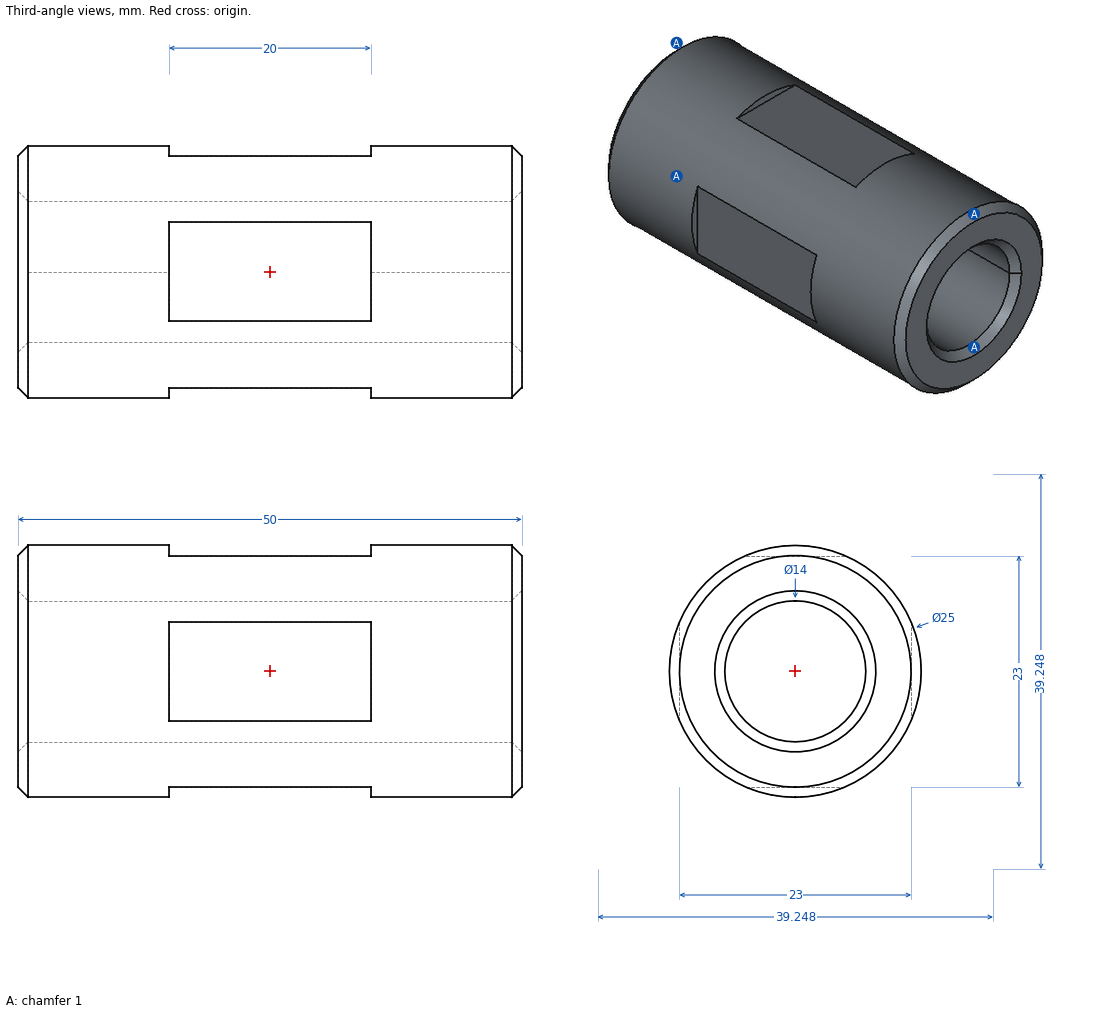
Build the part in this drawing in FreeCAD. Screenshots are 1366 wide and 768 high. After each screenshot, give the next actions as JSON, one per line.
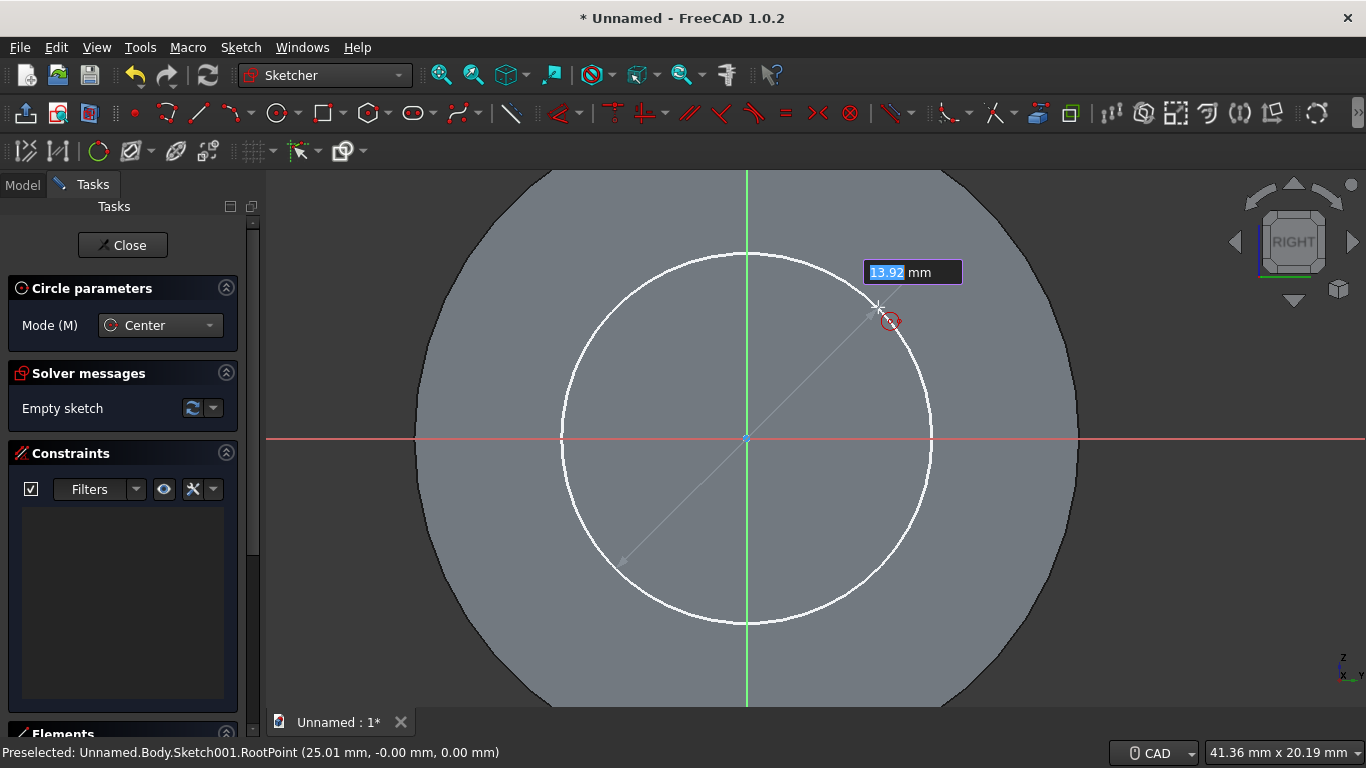
{"action": "type", "text": "14"}
{"action": "key", "text": "Return"}
{"action": "key", "text": "Escape"}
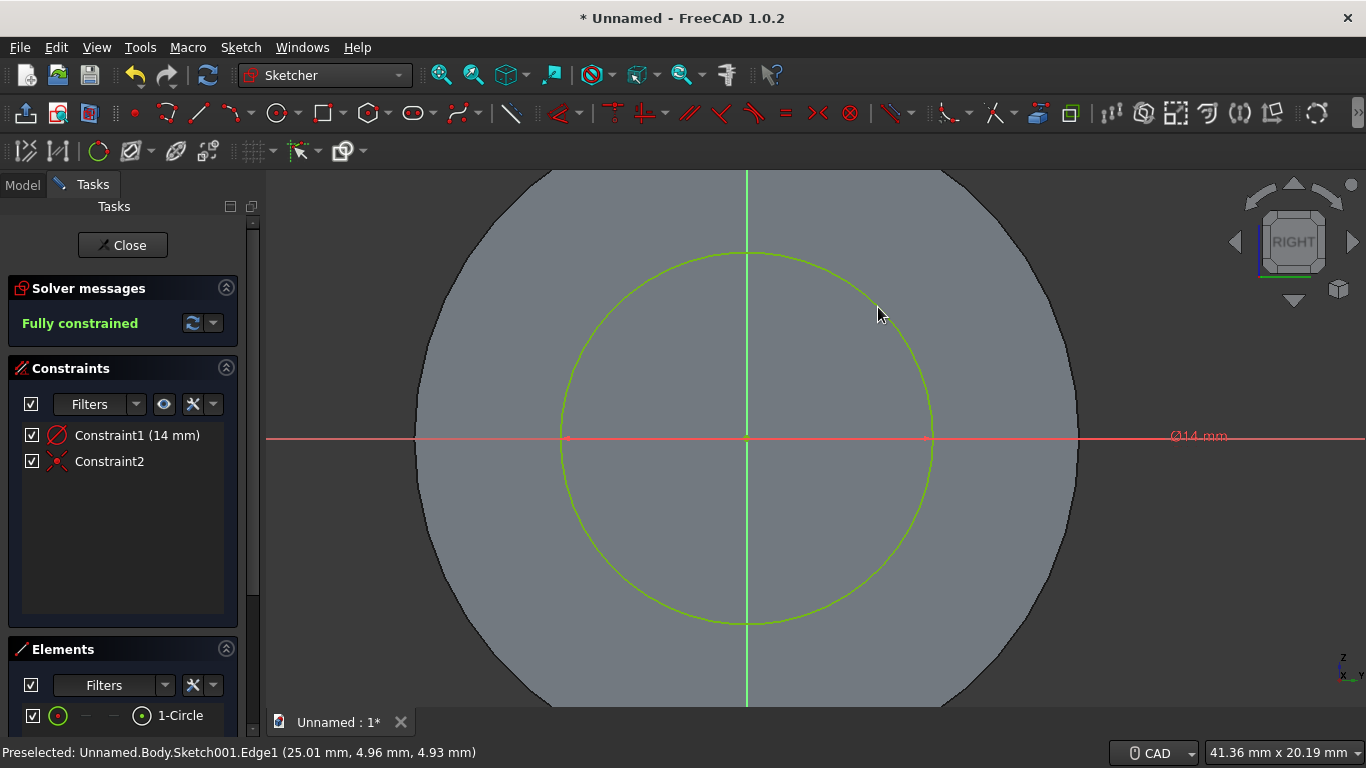
{"action": "left_click", "coordinate": [123, 245]}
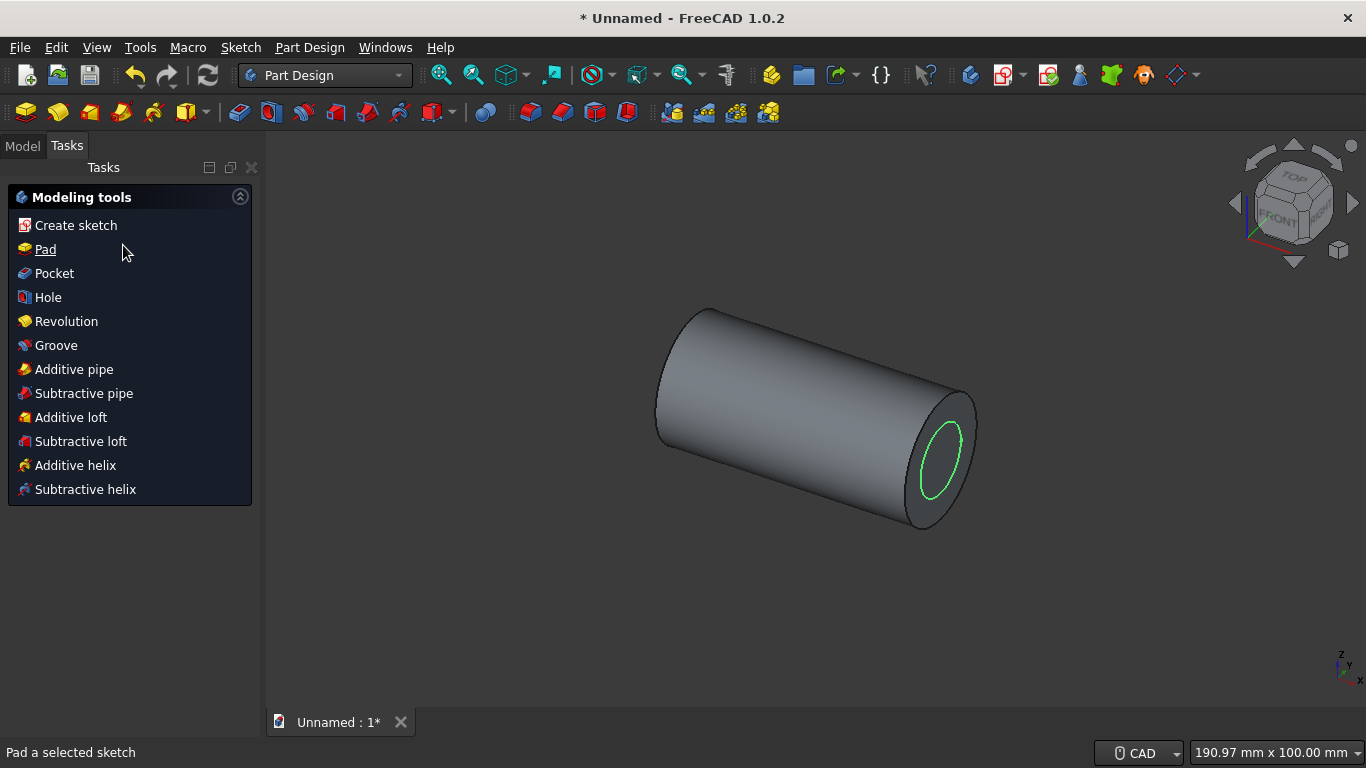
{"action": "left_click", "coordinate": [240, 112]}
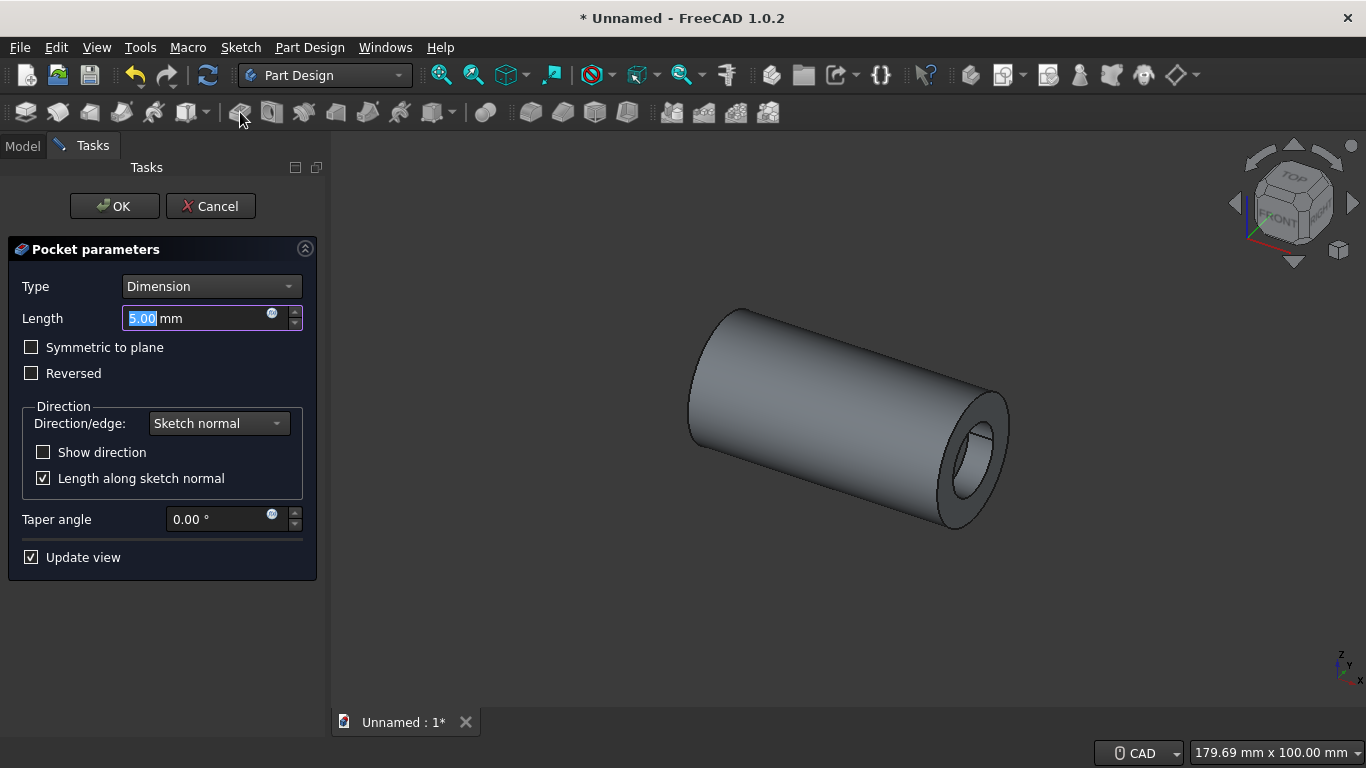
{"action": "left_click", "coordinate": [212, 286]}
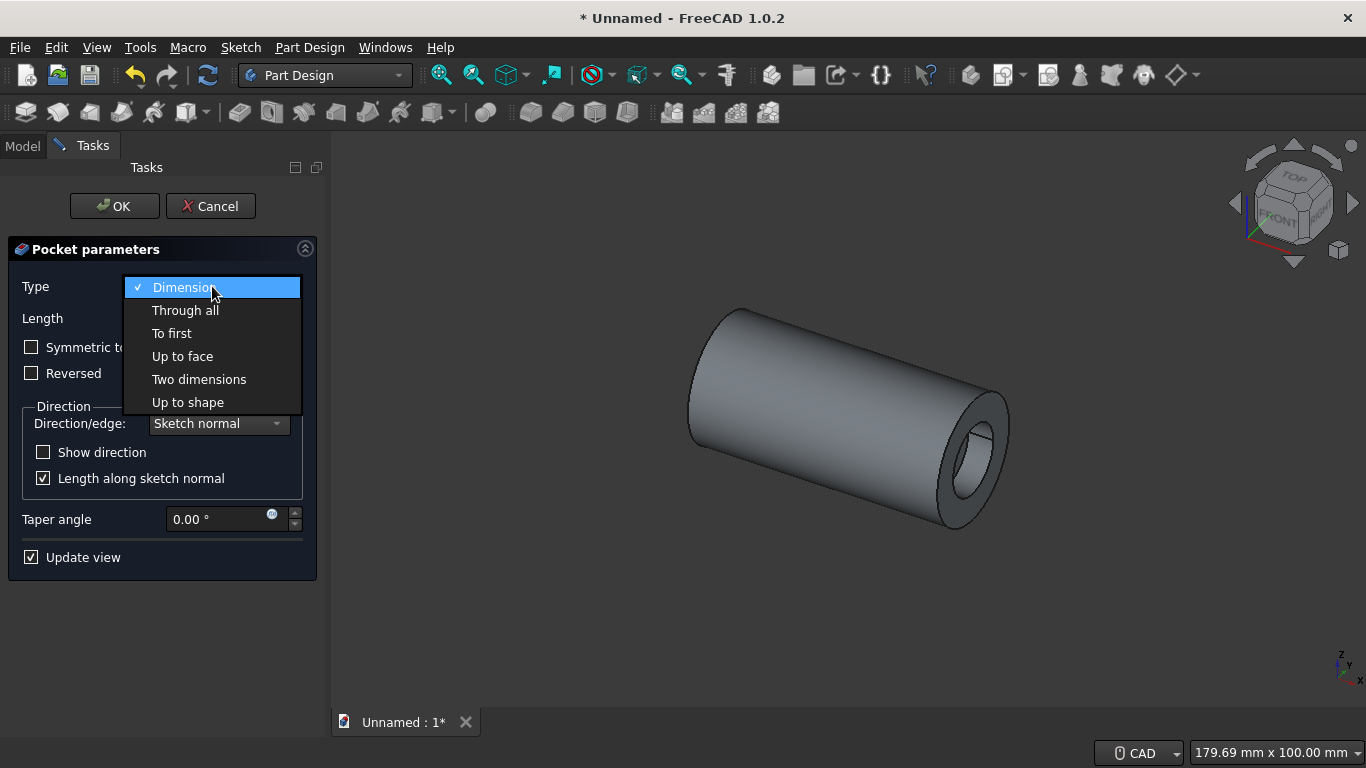
{"action": "left_click", "coordinate": [212, 310]}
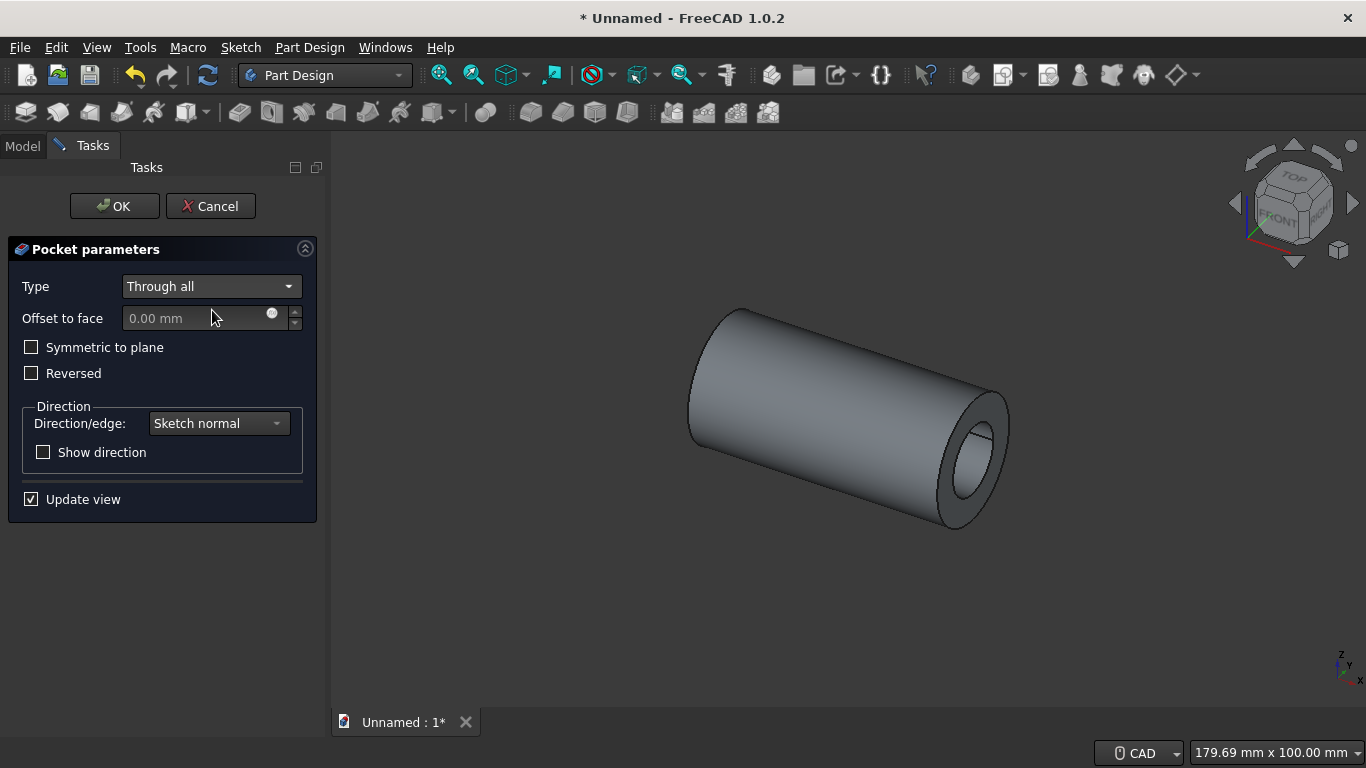
{"action": "left_click", "coordinate": [115, 206]}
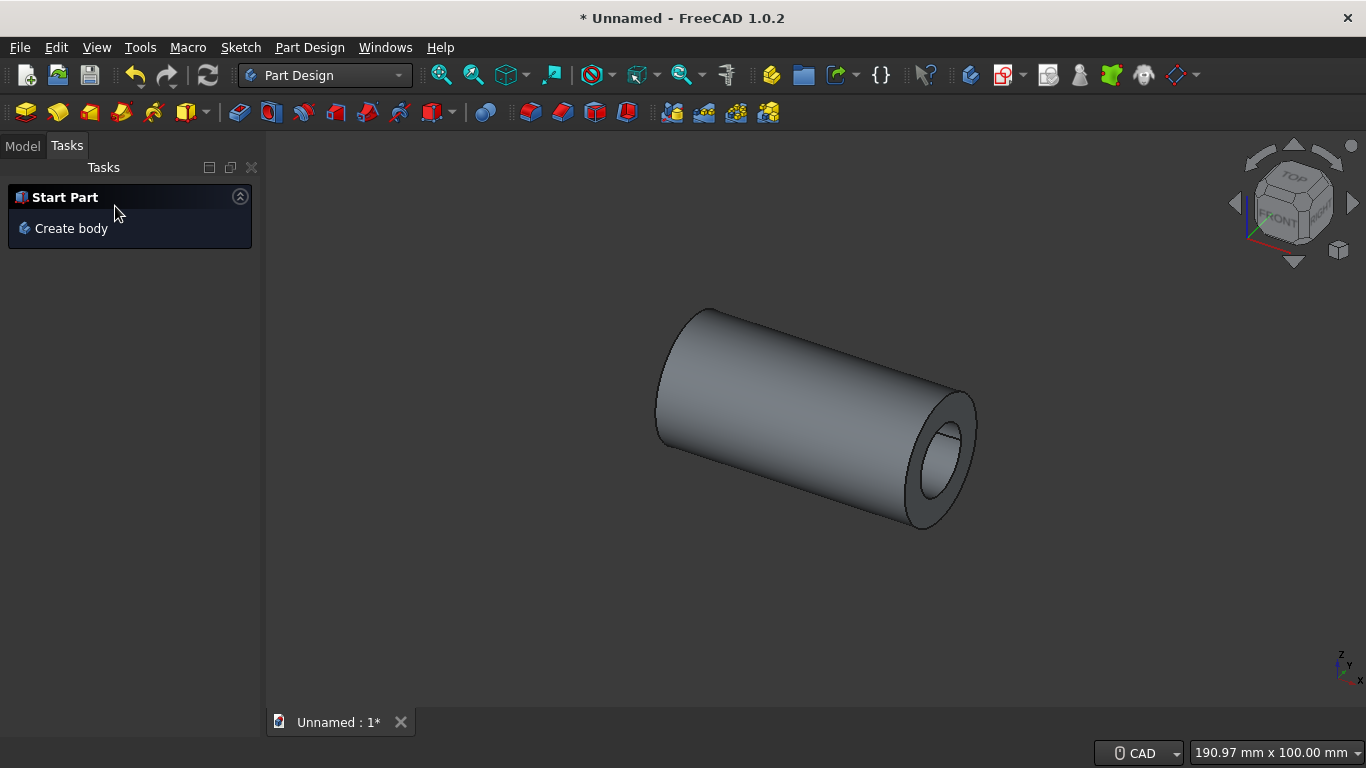
{"action": "left_click", "coordinate": [1004, 76]}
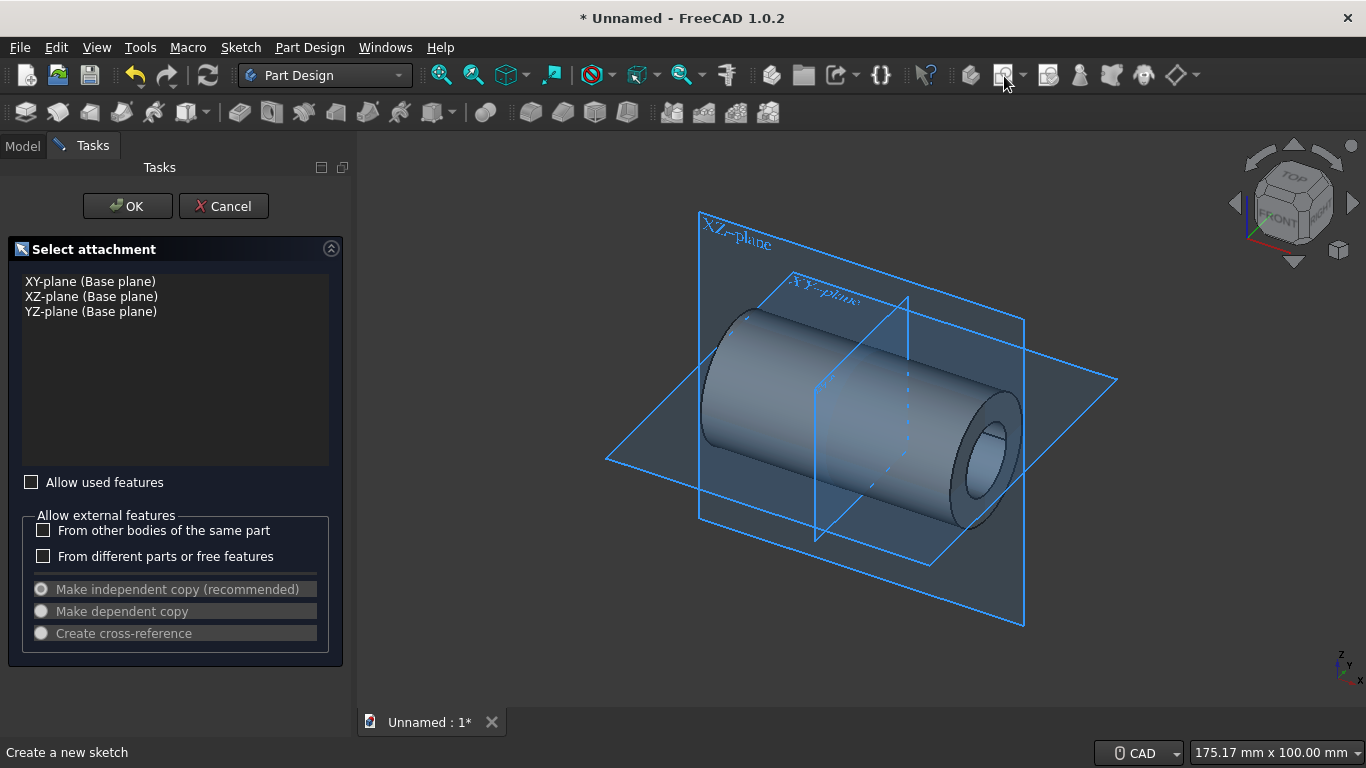
{"action": "left_click", "coordinate": [82, 312]}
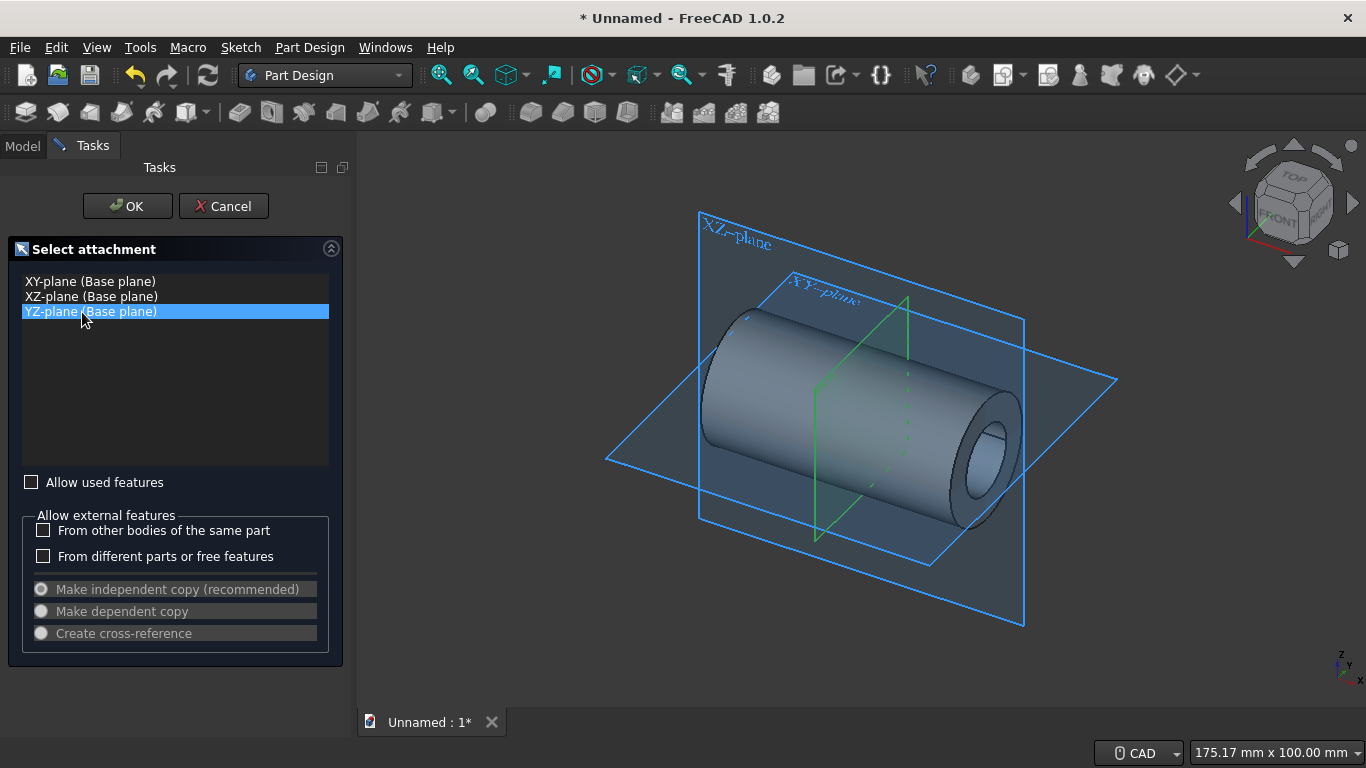
{"action": "left_click", "coordinate": [128, 206]}